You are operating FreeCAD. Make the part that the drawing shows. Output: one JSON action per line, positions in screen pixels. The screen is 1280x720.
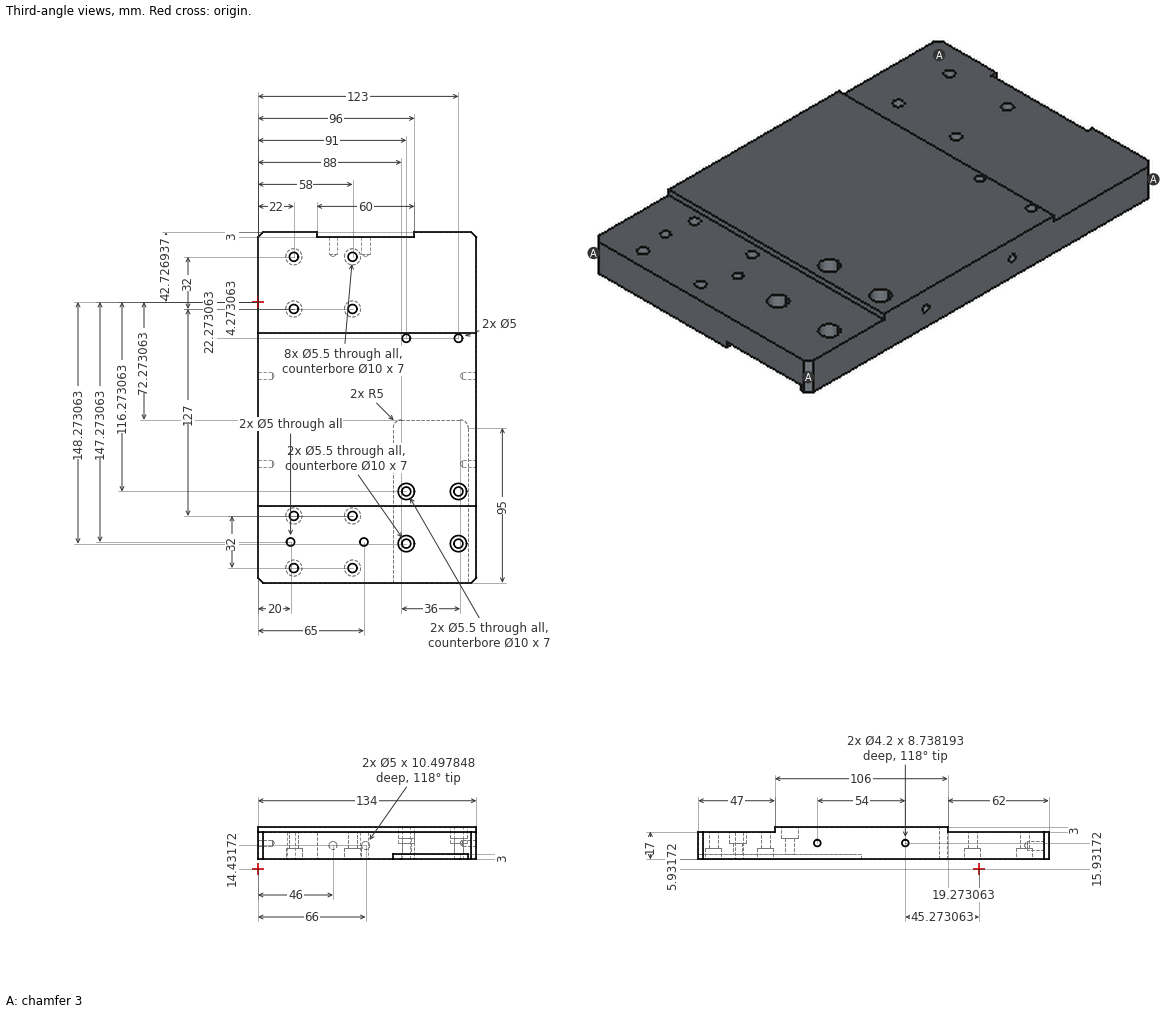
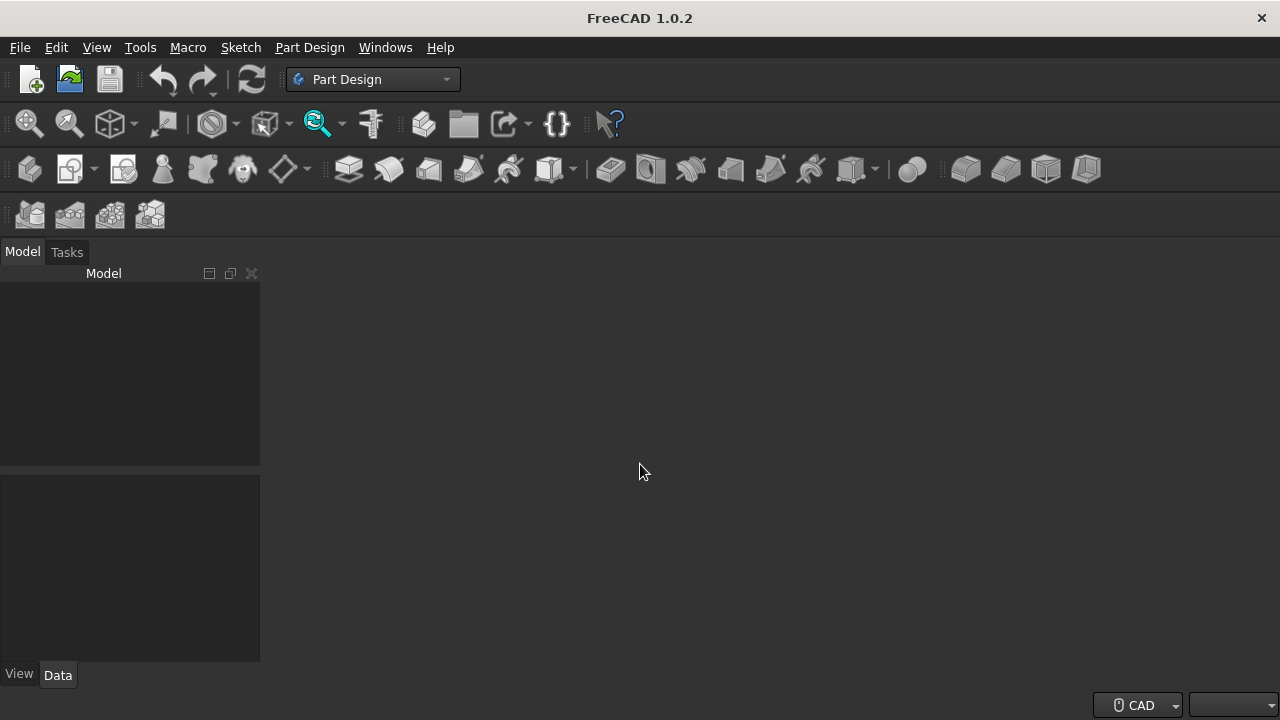
{"action": "left_click", "coordinate": [30, 80]}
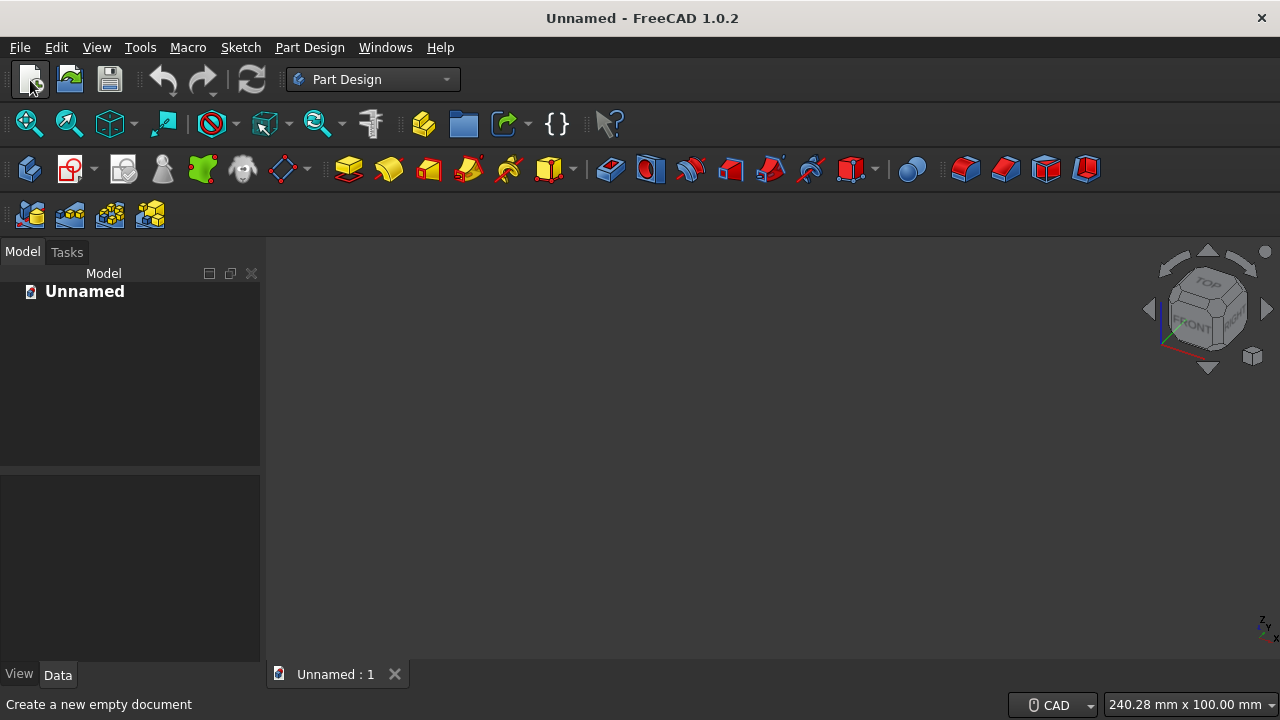
{"action": "left_click", "coordinate": [70, 170]}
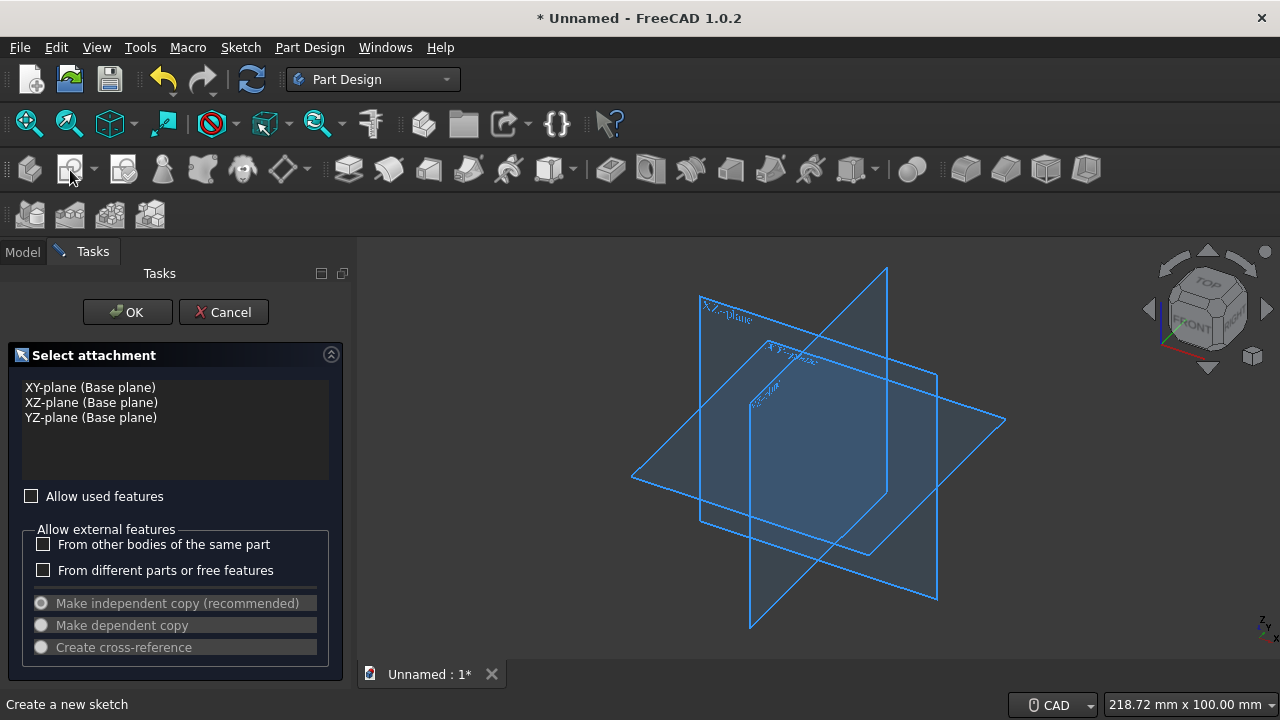
{"action": "left_click", "coordinate": [82, 418]}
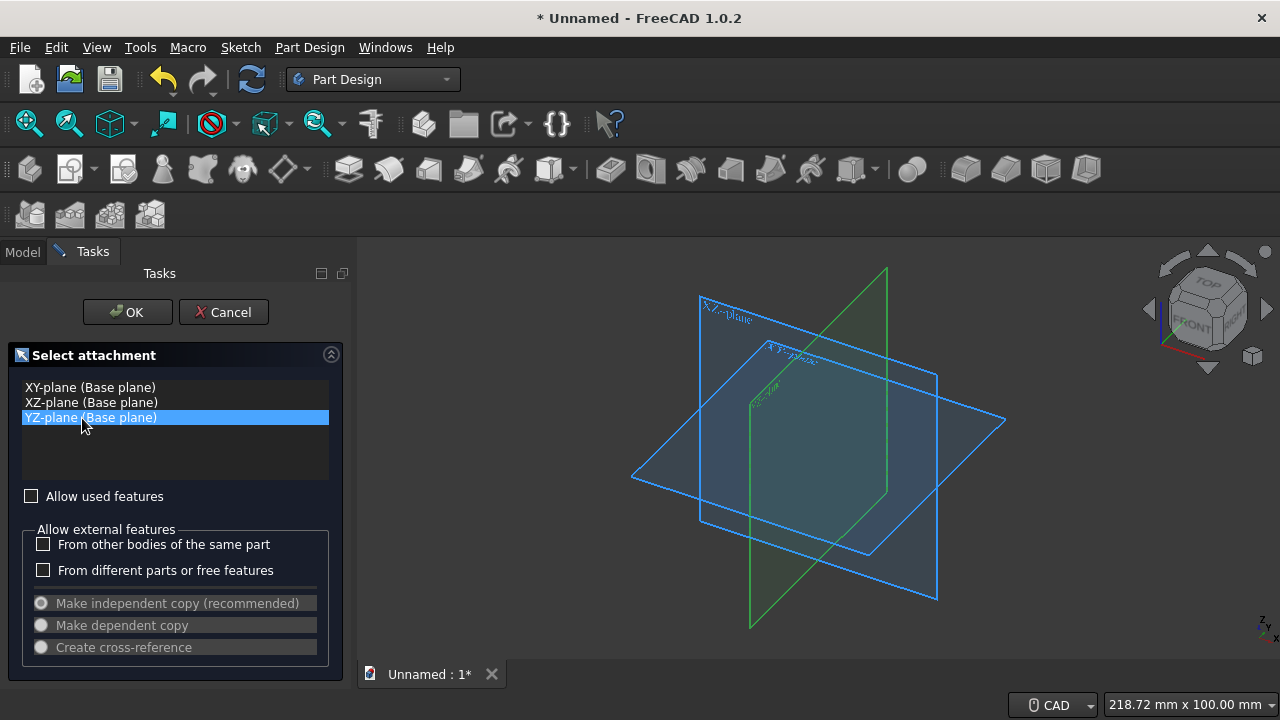
{"action": "left_click", "coordinate": [128, 312]}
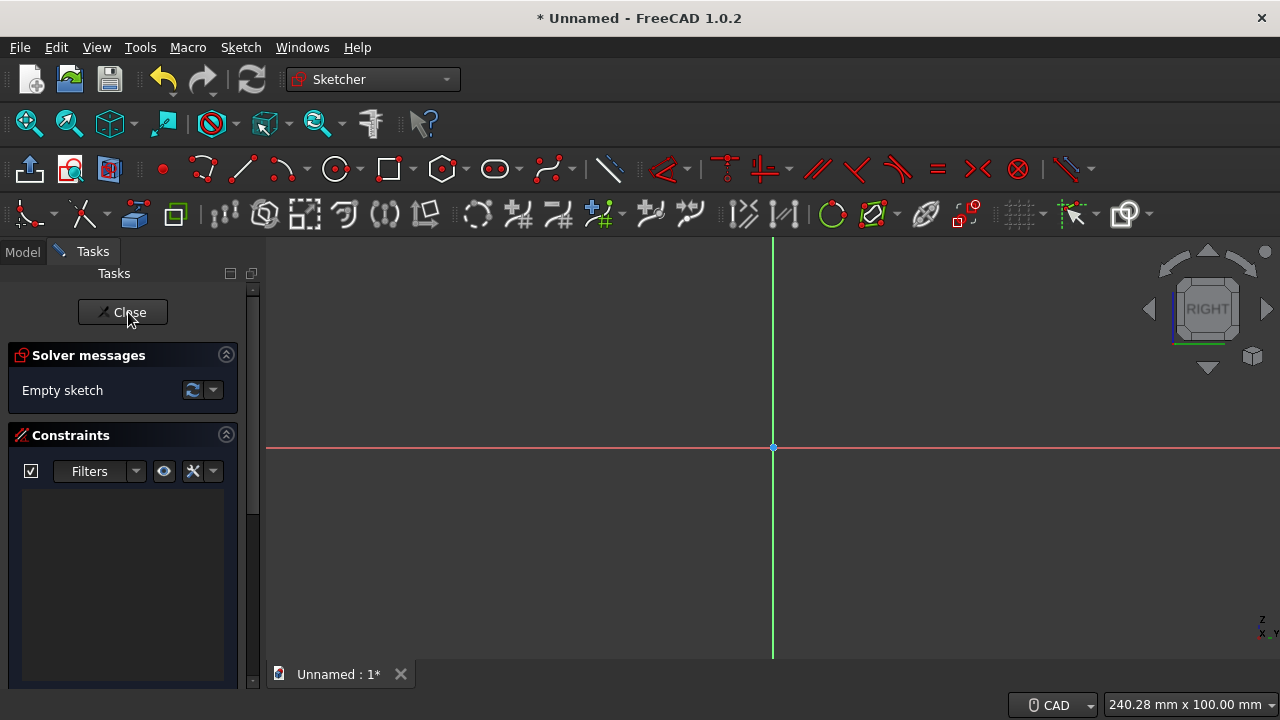
{"action": "scroll", "coordinate": [1115, 559], "scroll_direction": "down", "scroll_amount": 2}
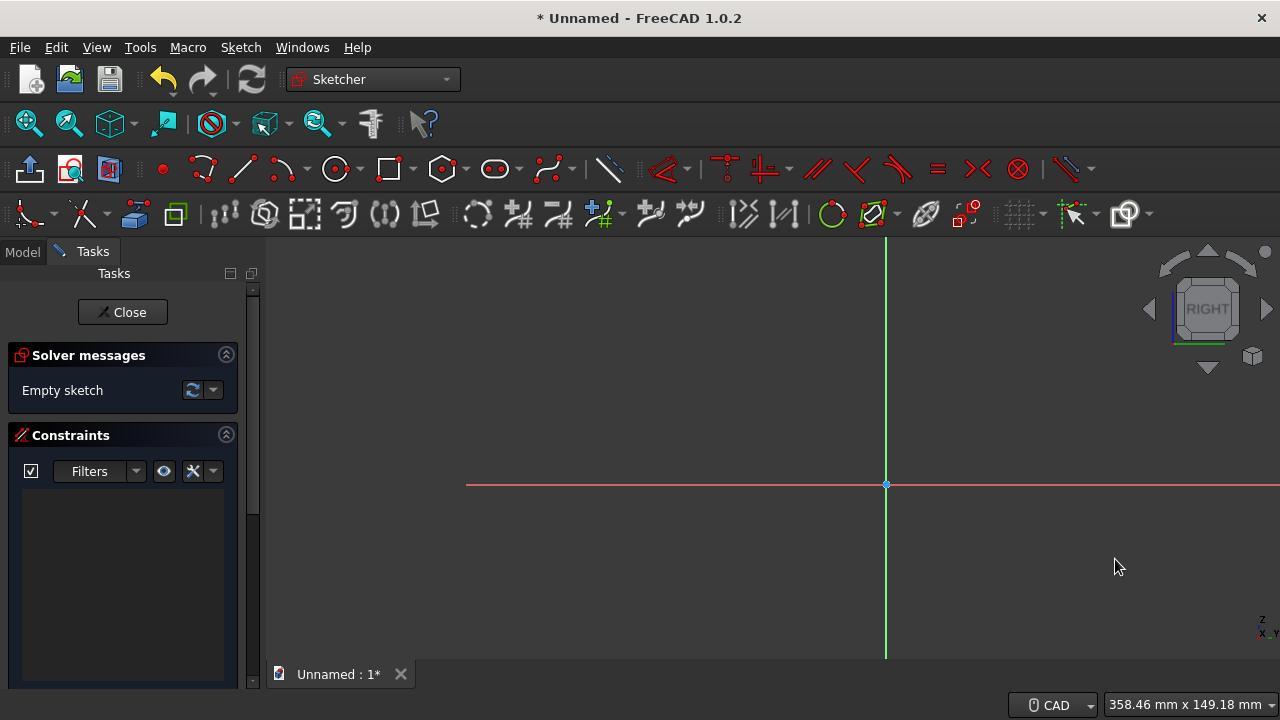
{"action": "left_click", "coordinate": [204, 170]}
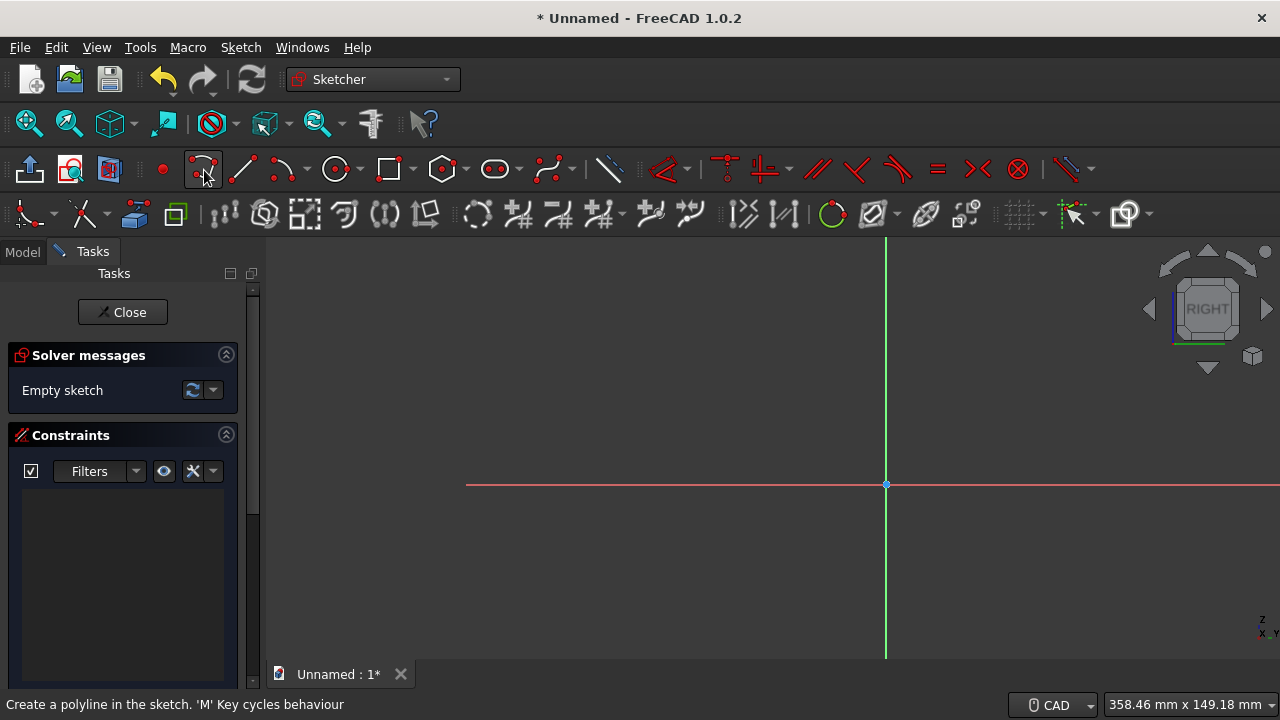
{"action": "left_click", "coordinate": [832, 420]}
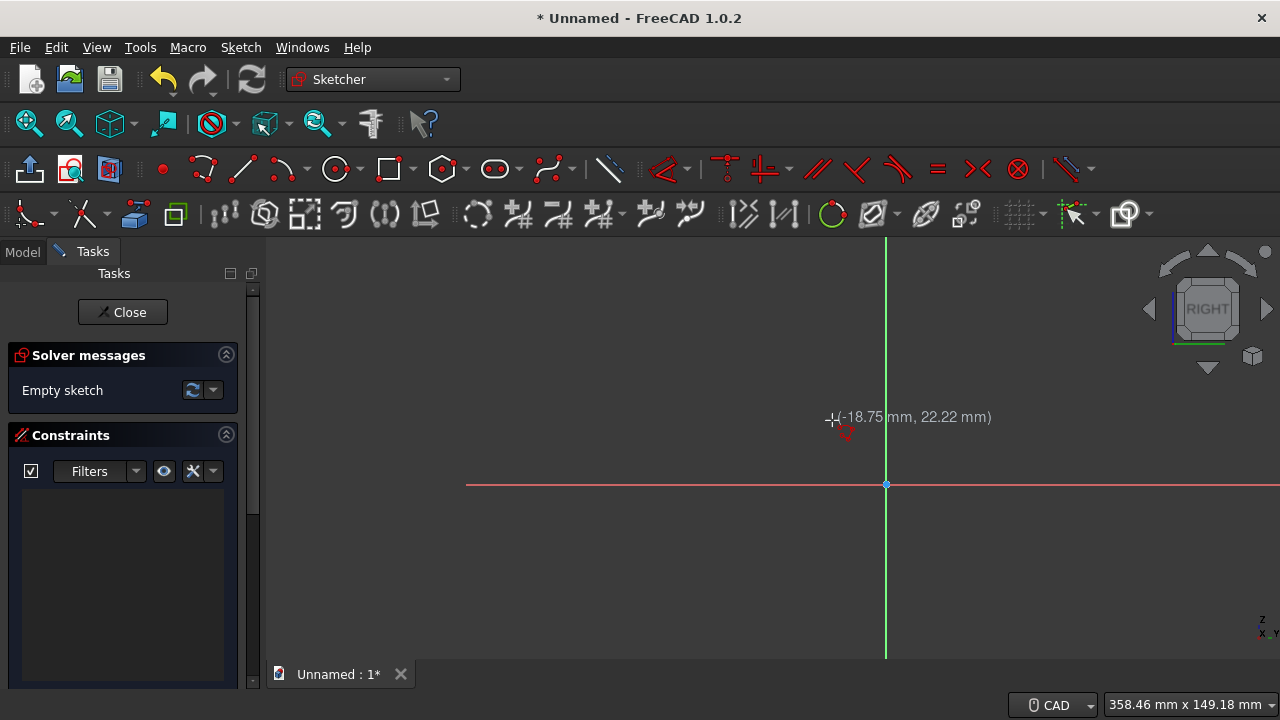
{"action": "scroll", "coordinate": [832, 411], "scroll_direction": "up", "scroll_amount": 4}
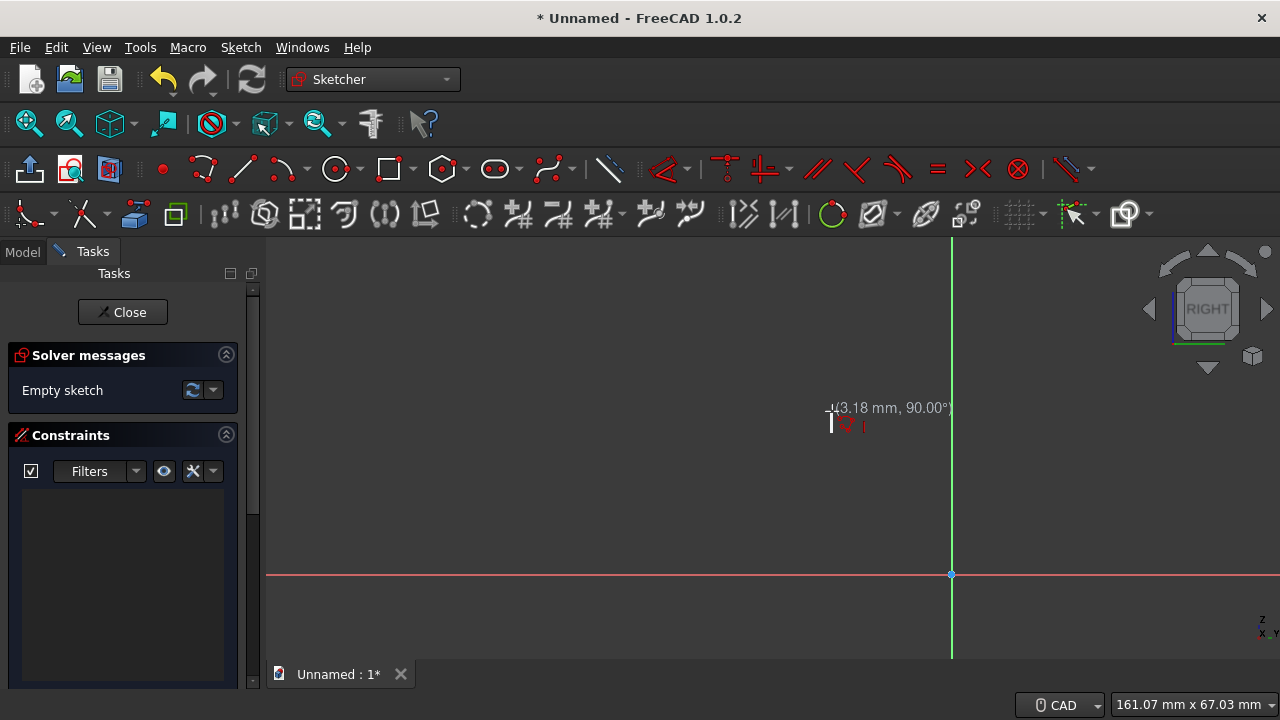
{"action": "left_click", "coordinate": [831, 412]}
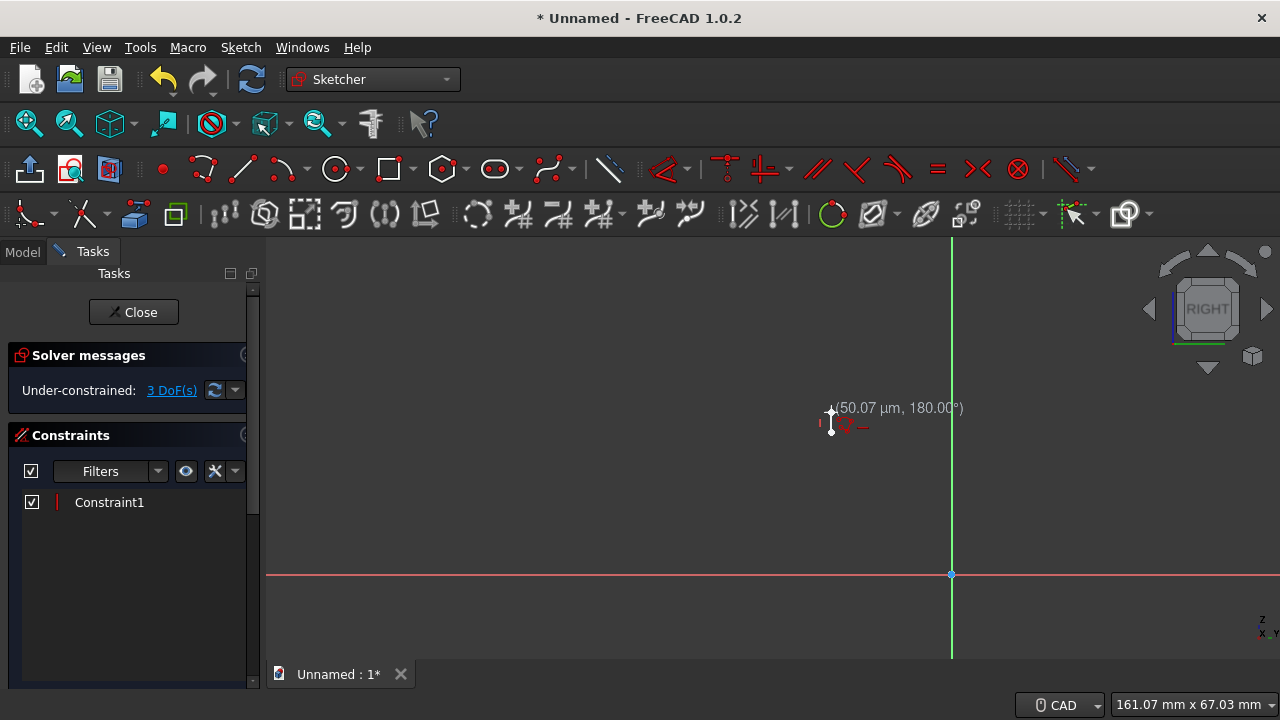
{"action": "scroll", "coordinate": [836, 411], "scroll_direction": "down", "scroll_amount": 4}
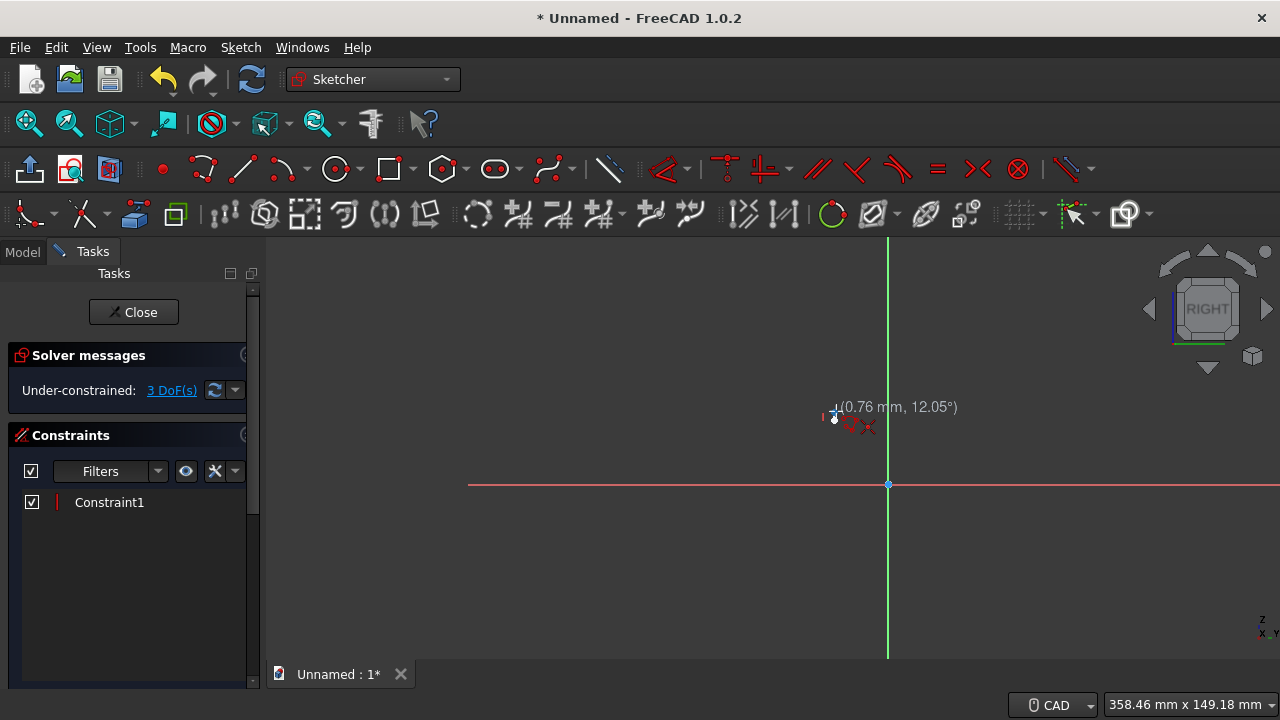
{"action": "left_click", "coordinate": [534, 412]}